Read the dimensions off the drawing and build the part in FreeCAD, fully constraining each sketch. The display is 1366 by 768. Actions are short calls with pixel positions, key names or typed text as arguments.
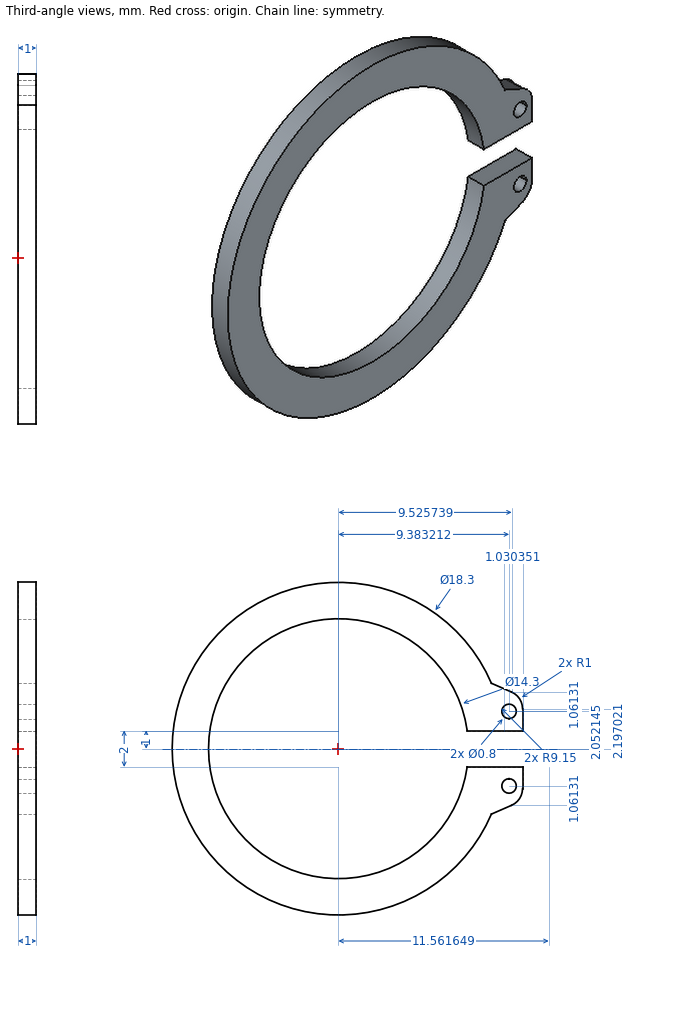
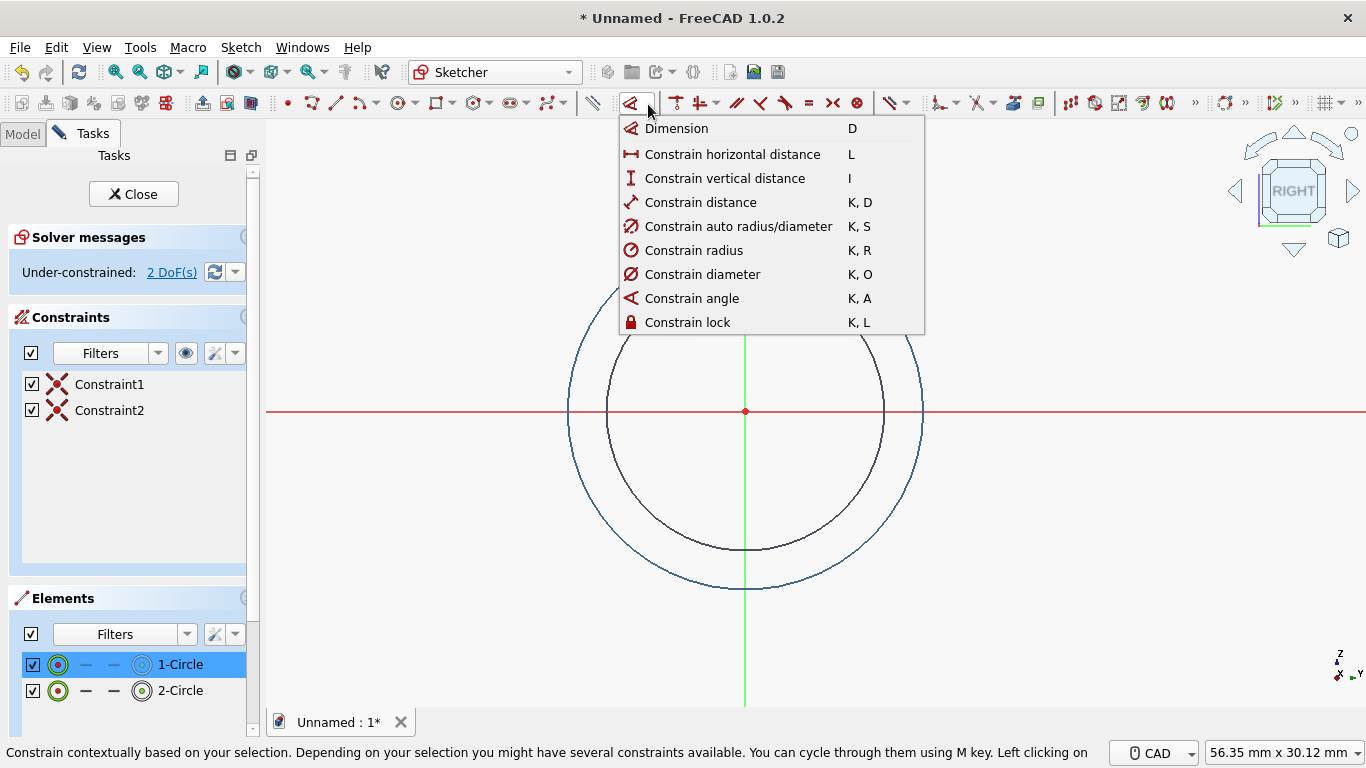
click(772, 274)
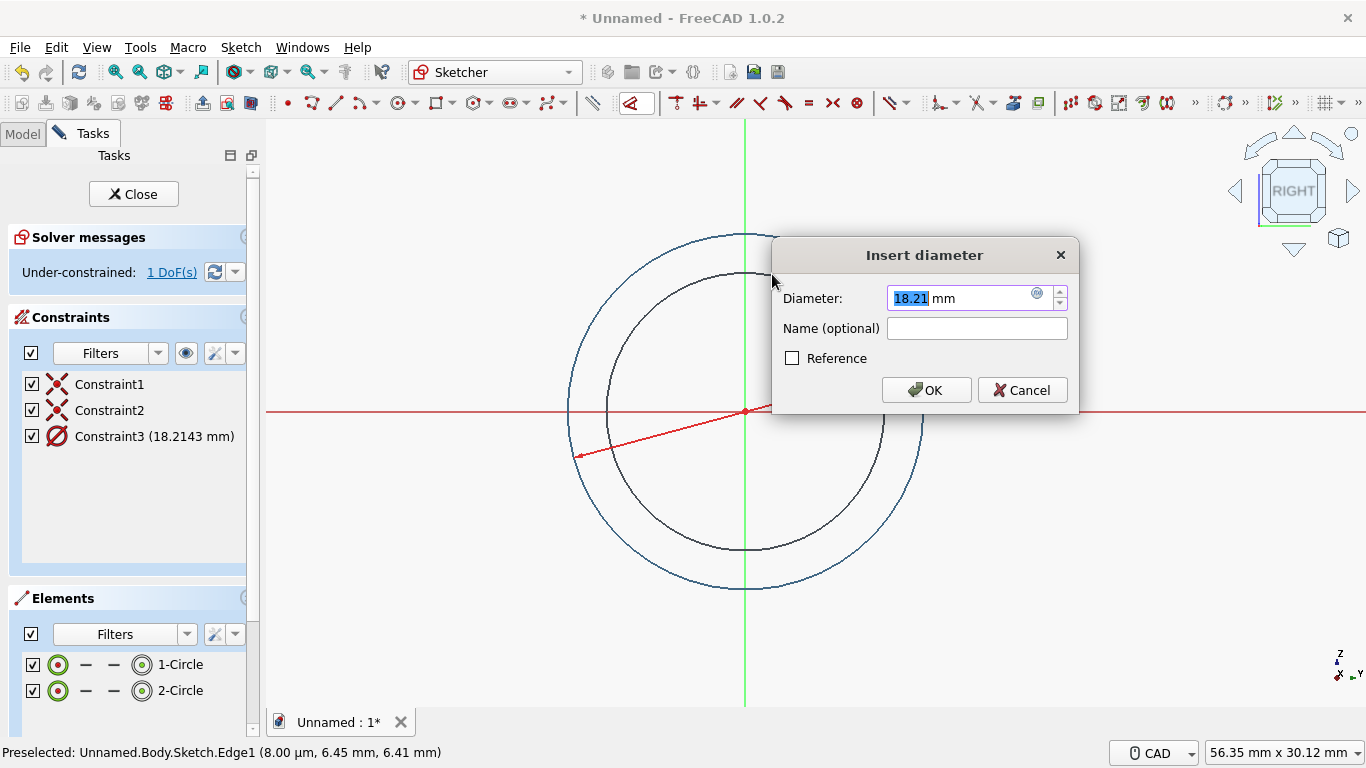
text(18.3)
key(Return)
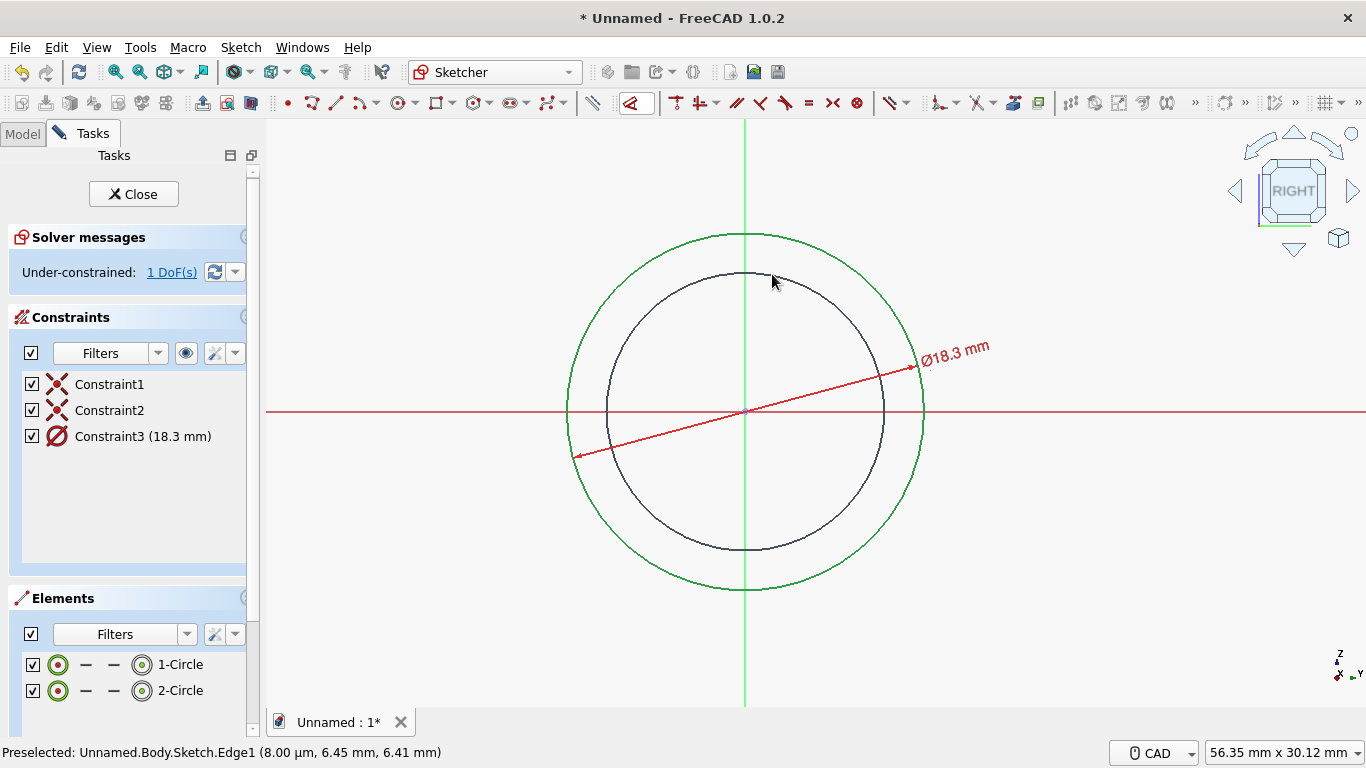
click(843, 313)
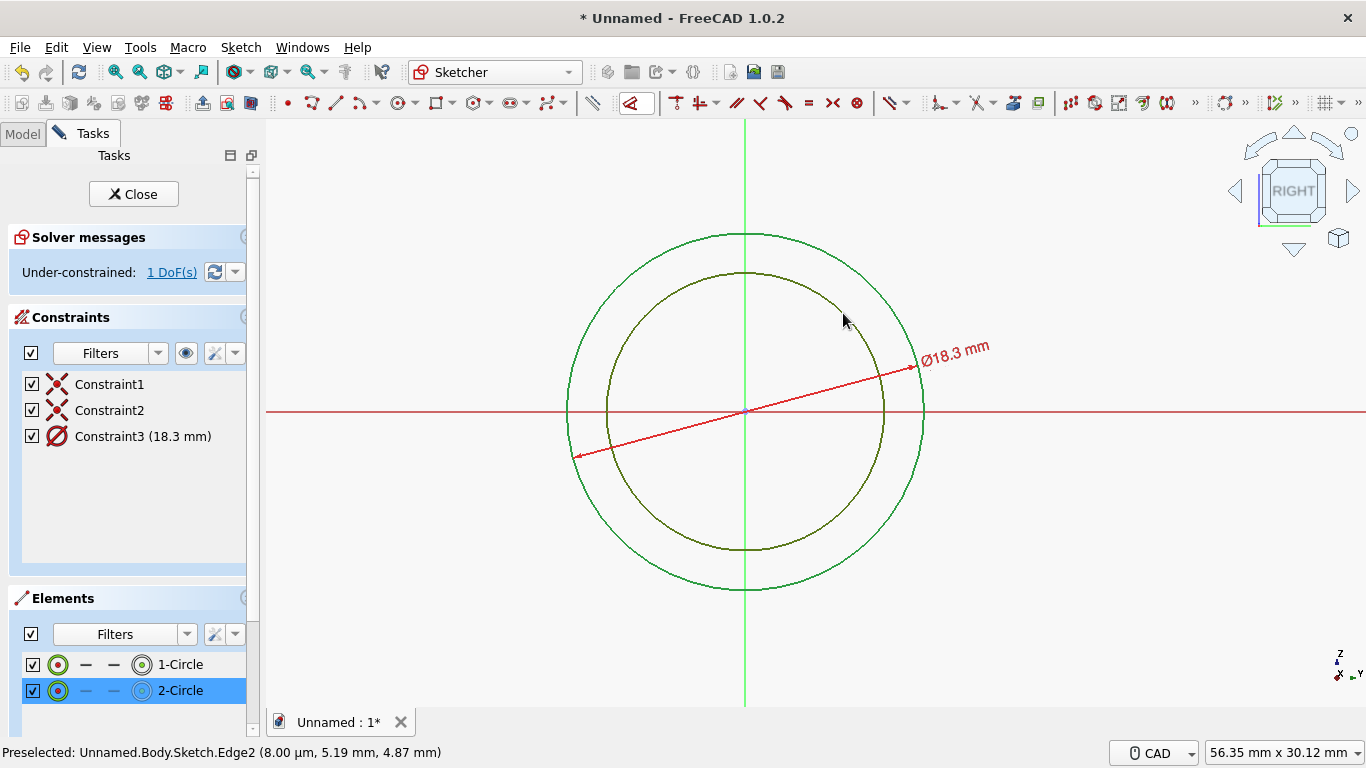
key(k)
key(o)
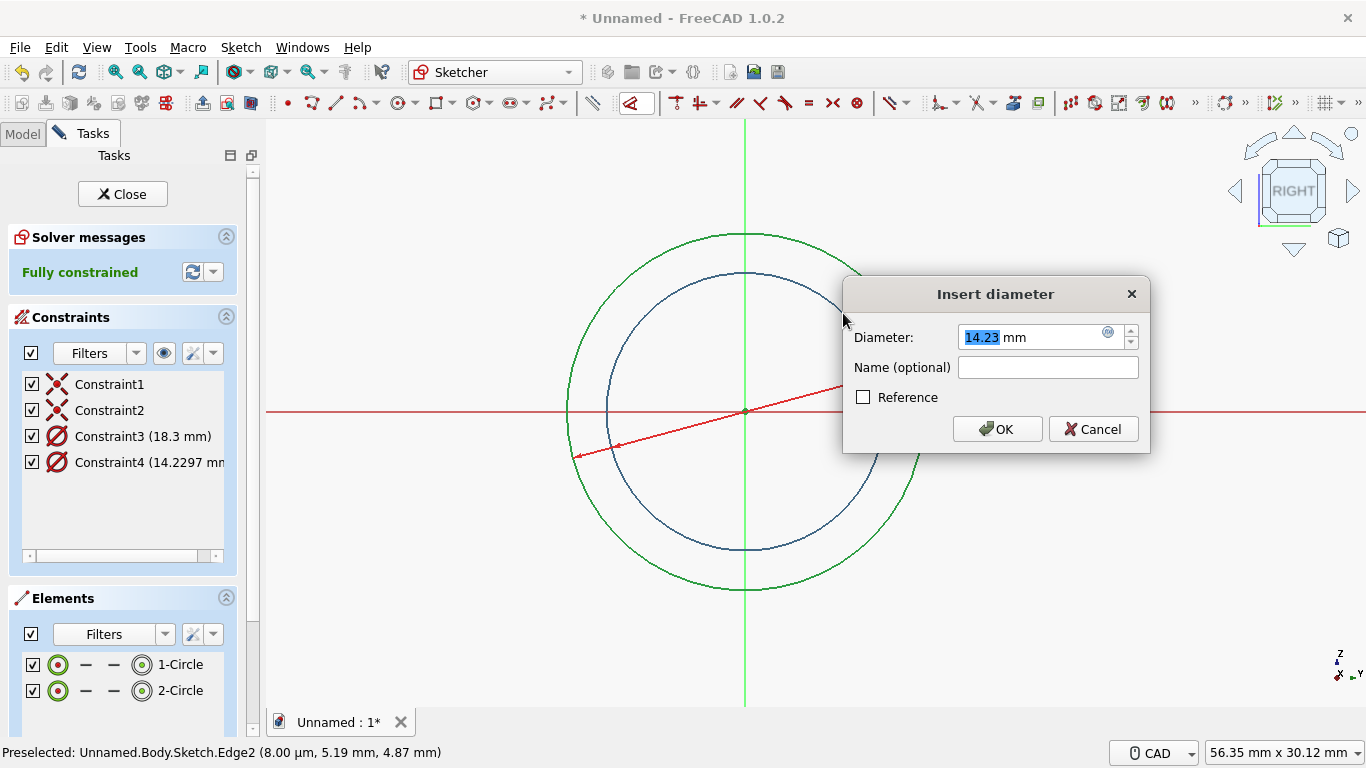
text(14.3)
key(Return)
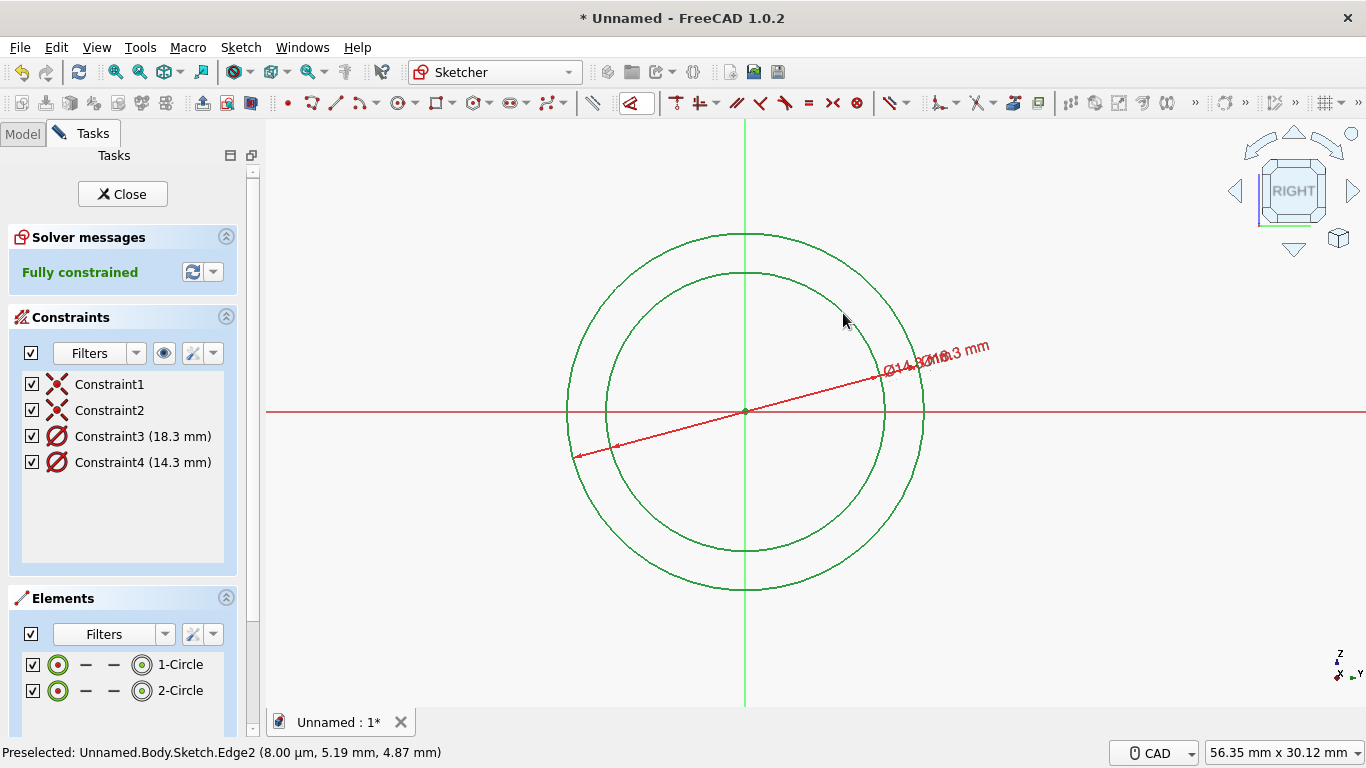
click(123, 194)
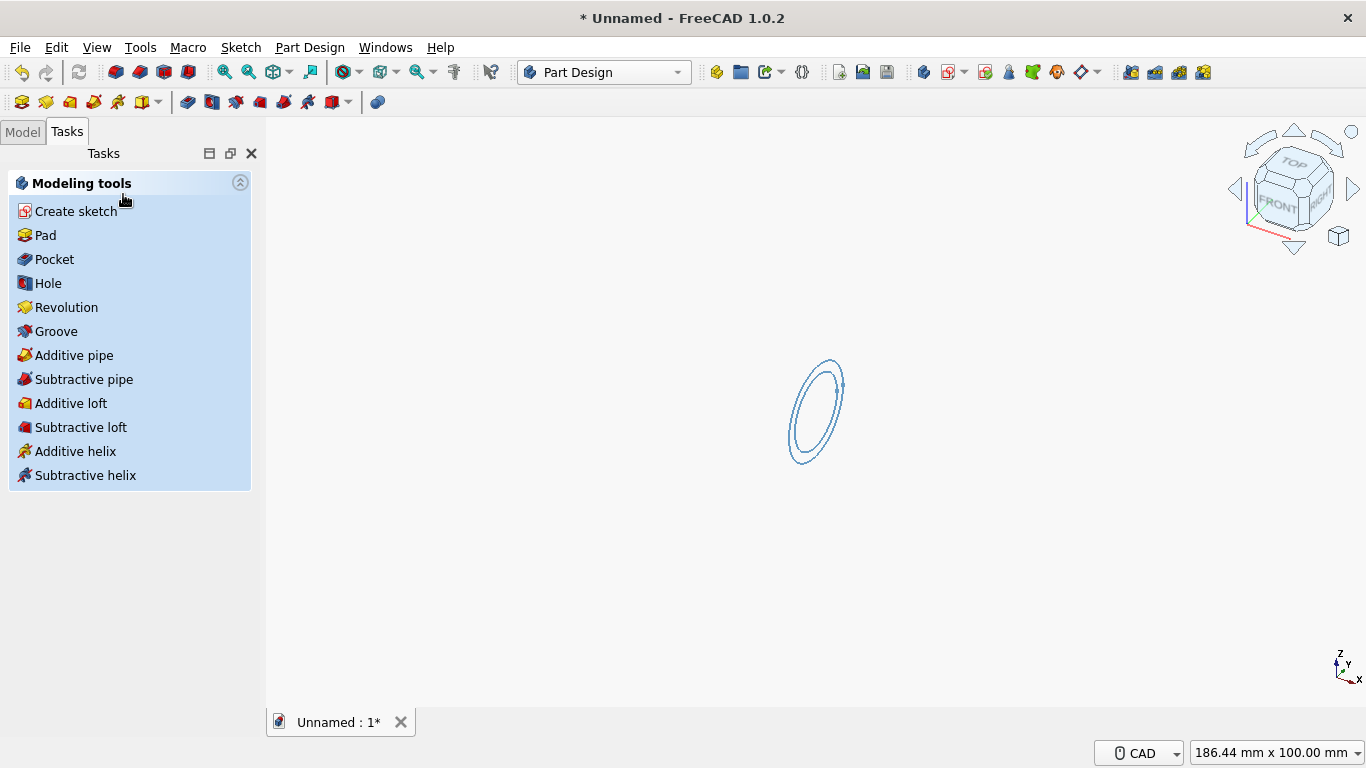
click(22, 102)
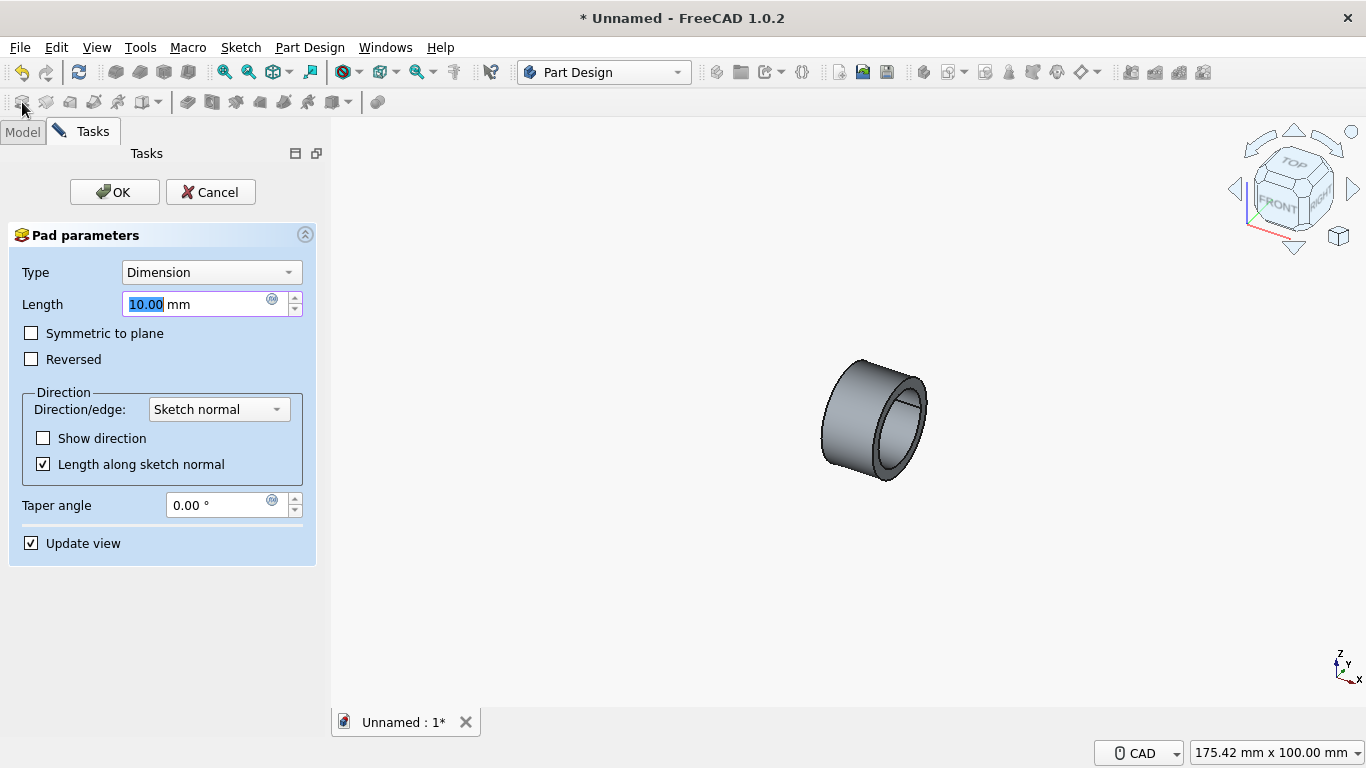
text(1)
key(Tab)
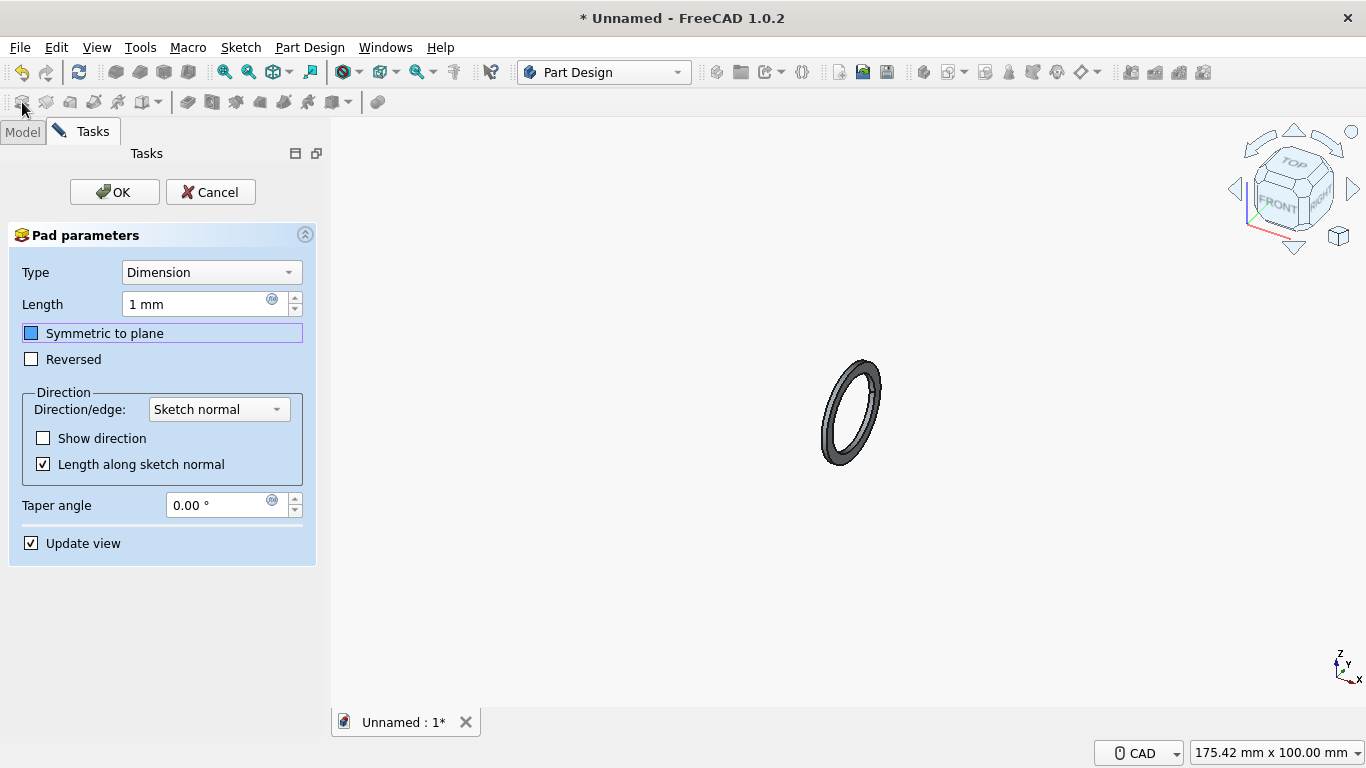
click(115, 192)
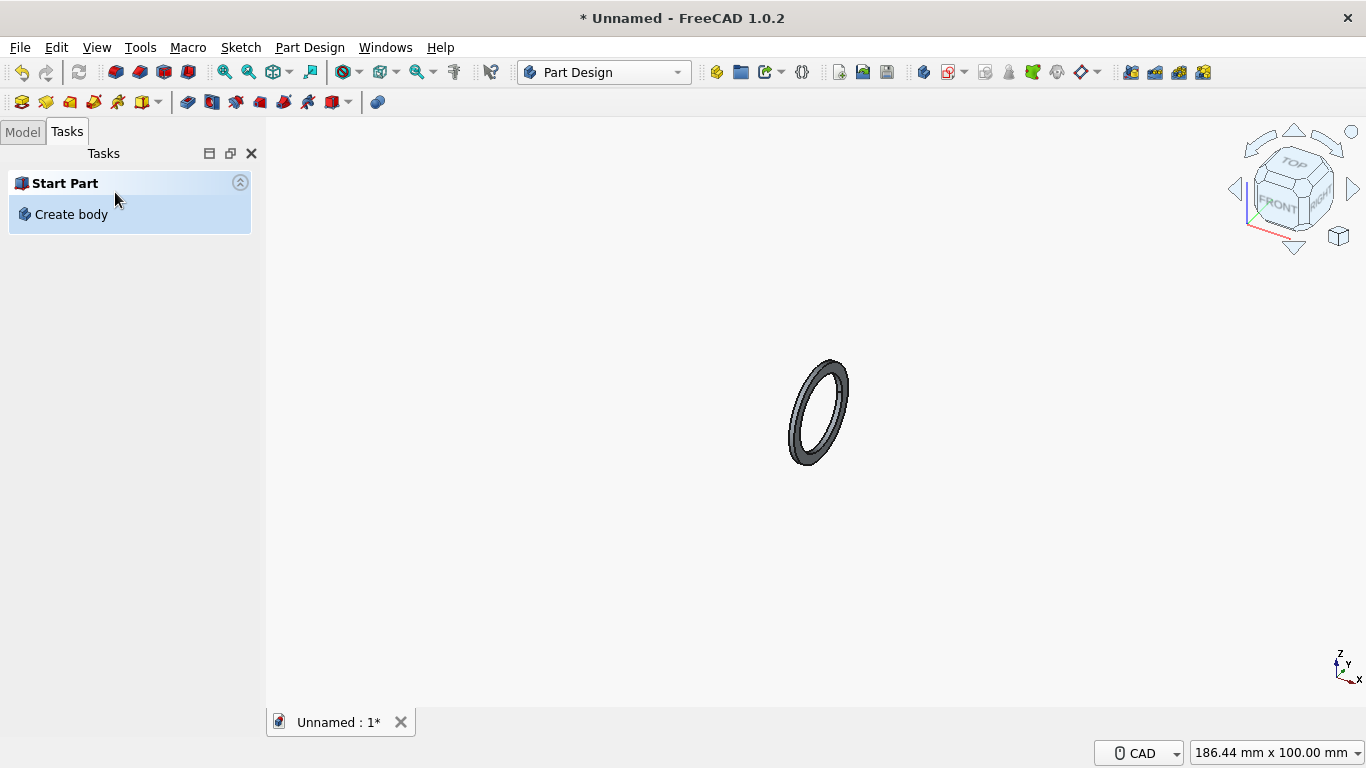
key(v)
key(f)